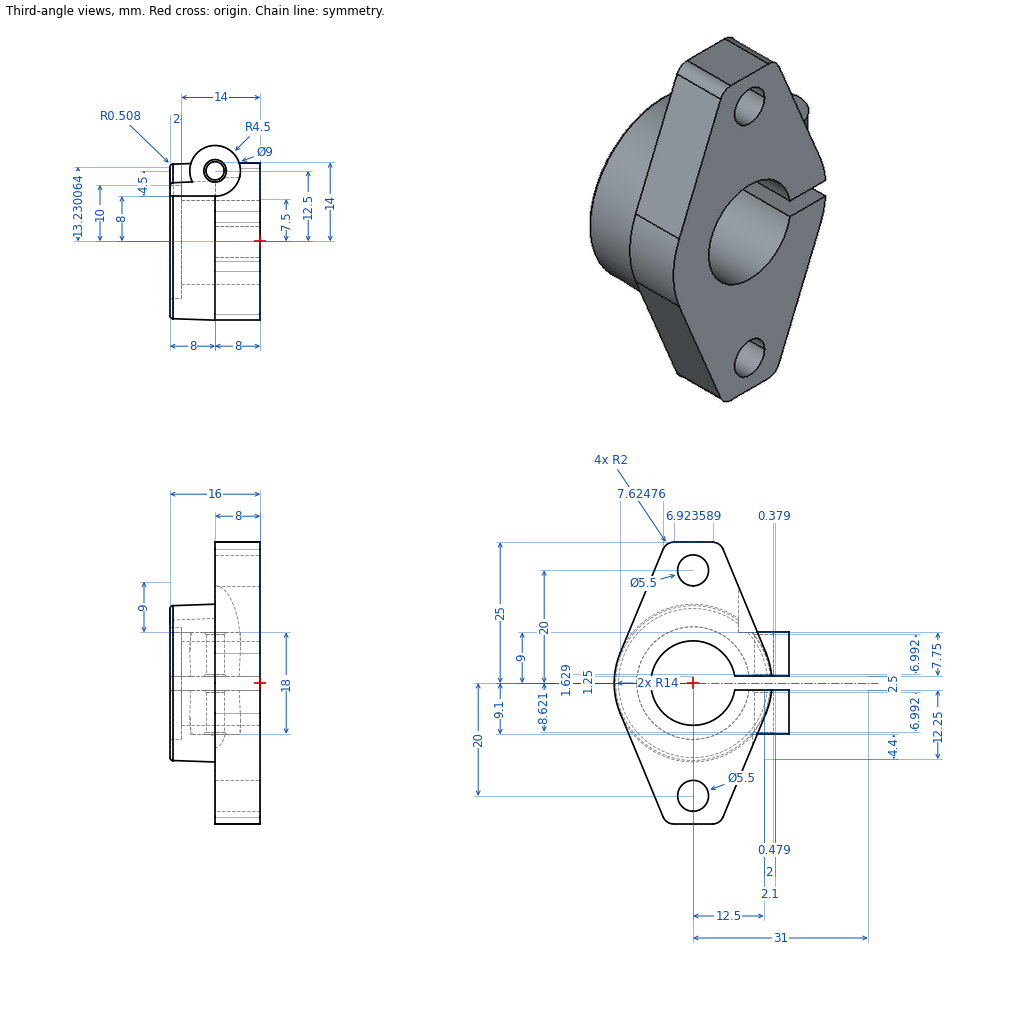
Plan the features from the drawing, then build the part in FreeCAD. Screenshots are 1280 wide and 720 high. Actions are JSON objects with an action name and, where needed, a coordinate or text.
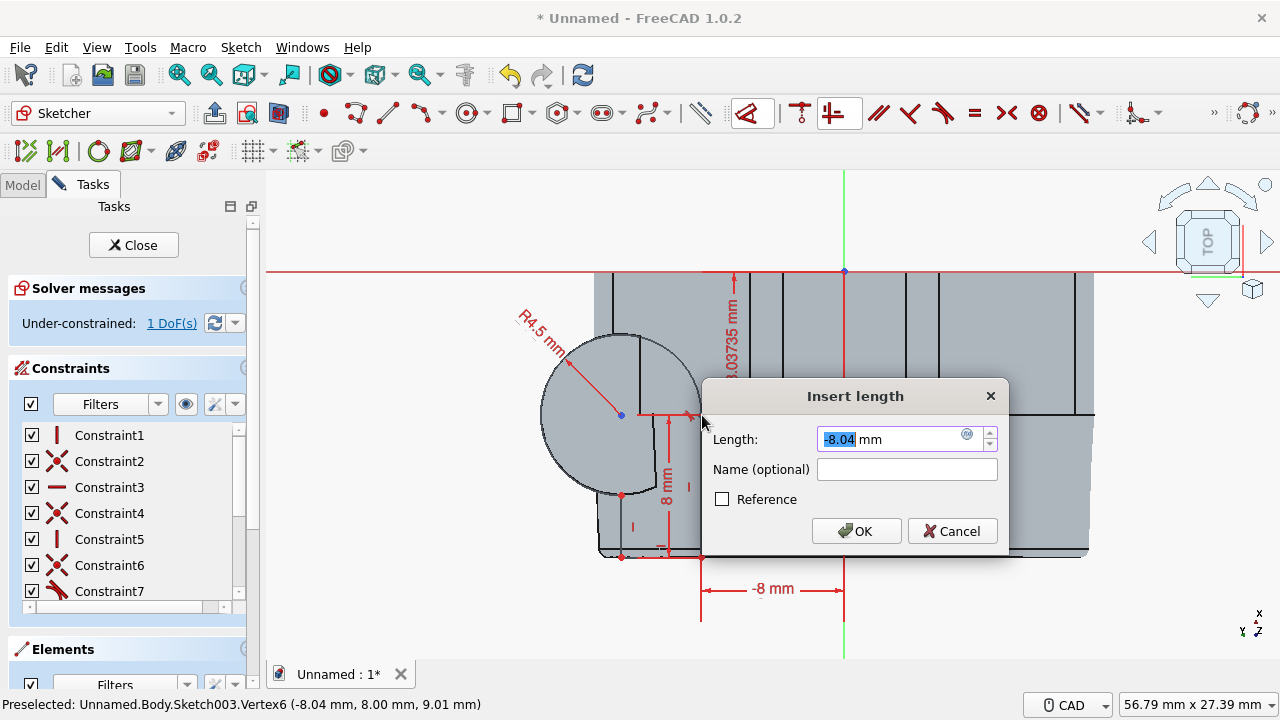
{"action": "type", "text": "-8"}
{"action": "key", "text": "Return"}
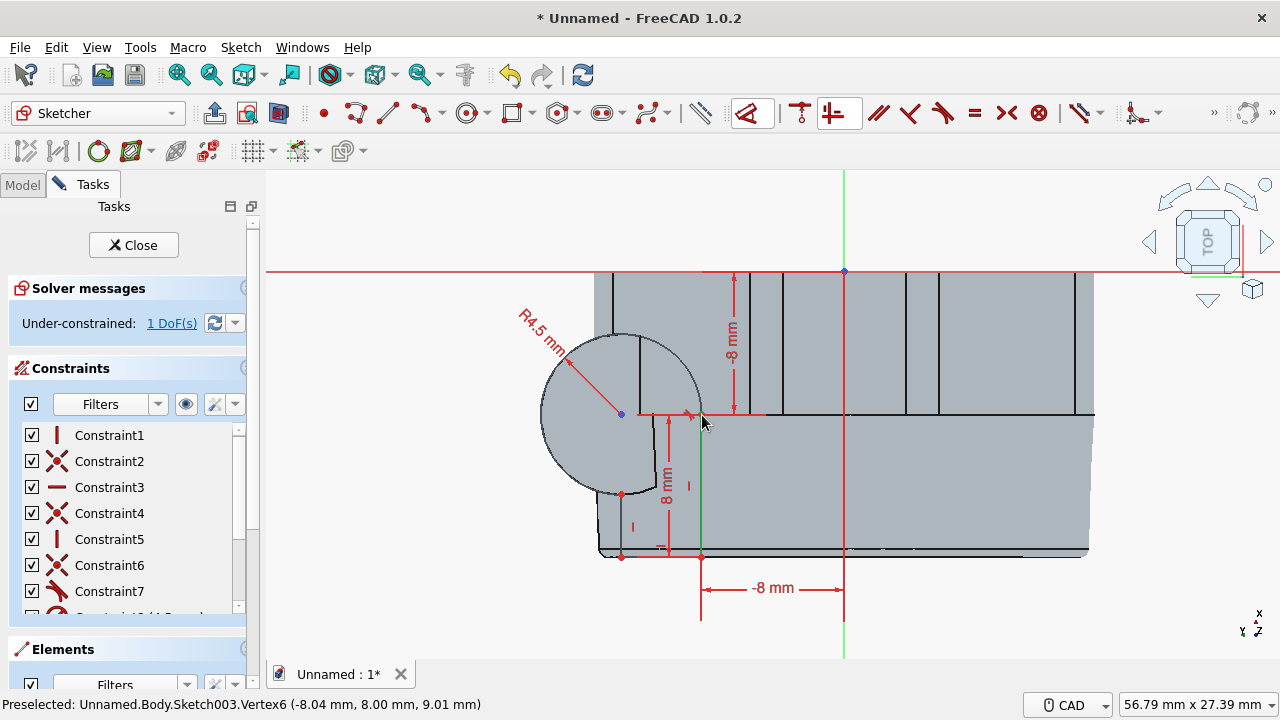
{"action": "left_click", "coordinate": [645, 557]}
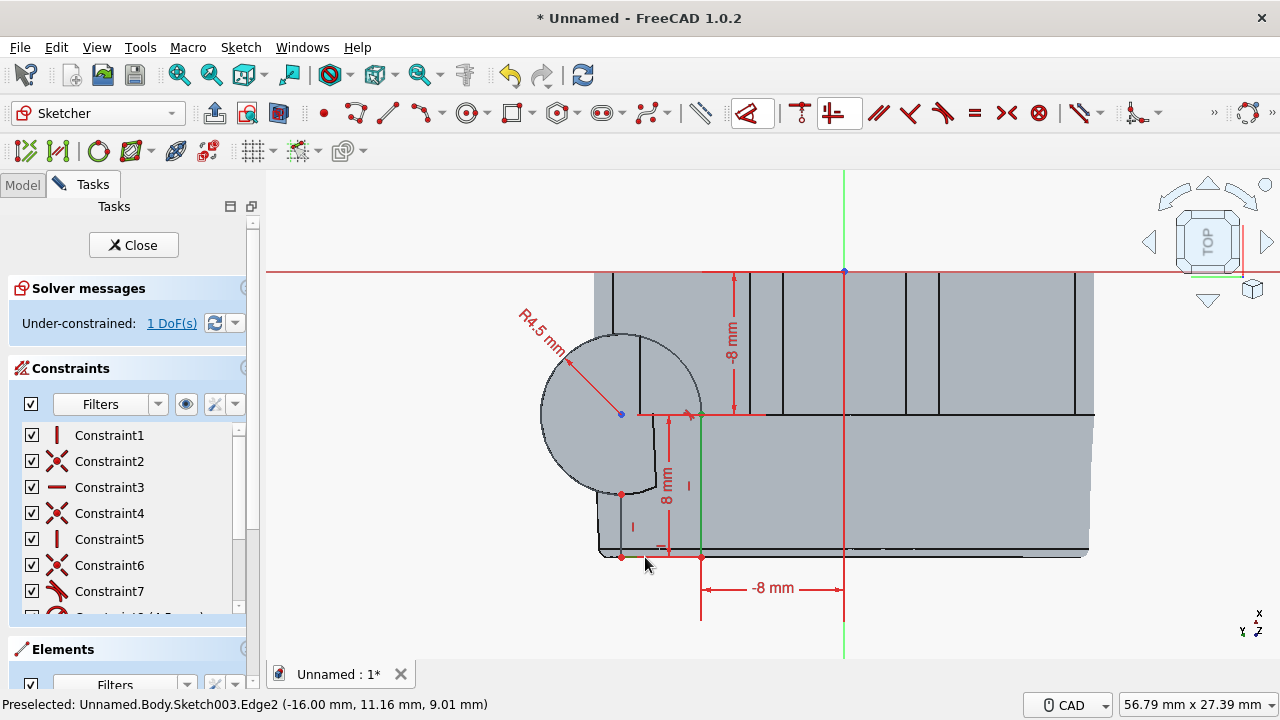
{"action": "left_click", "coordinate": [768, 114]}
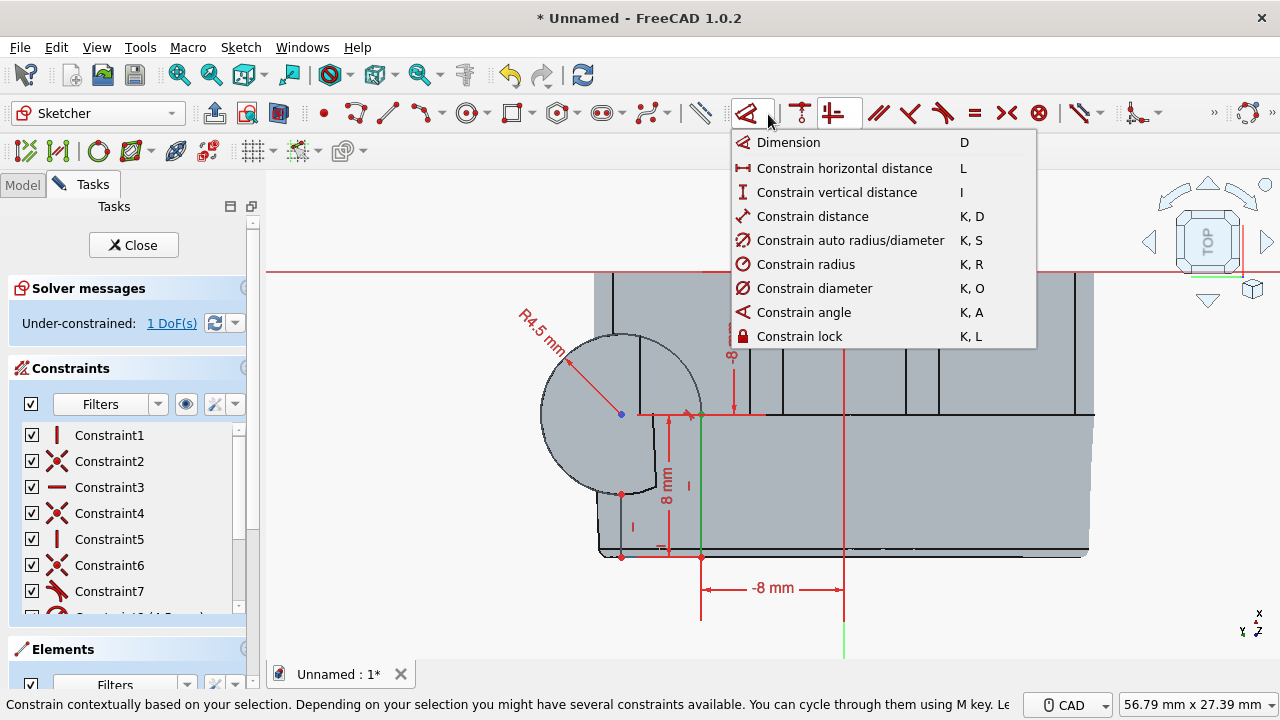
{"action": "left_click", "coordinate": [884, 168]}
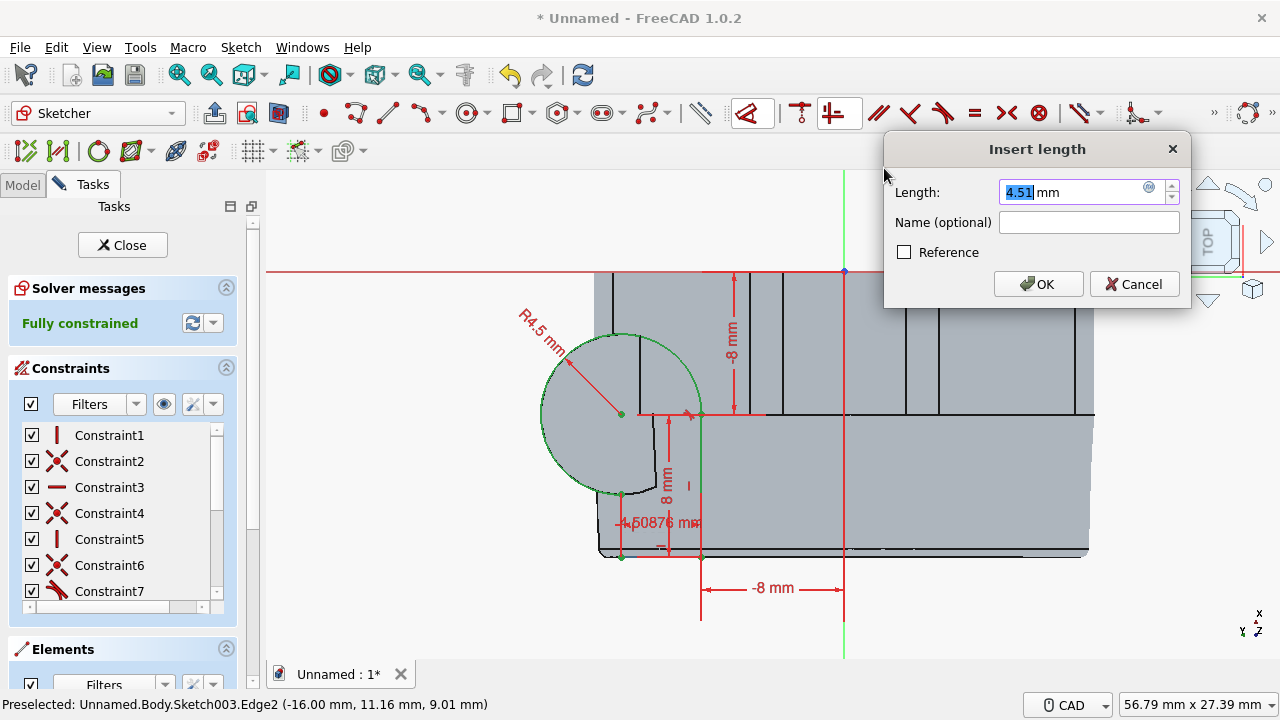
{"action": "type", "text": "4.5"}
{"action": "key", "text": "Return"}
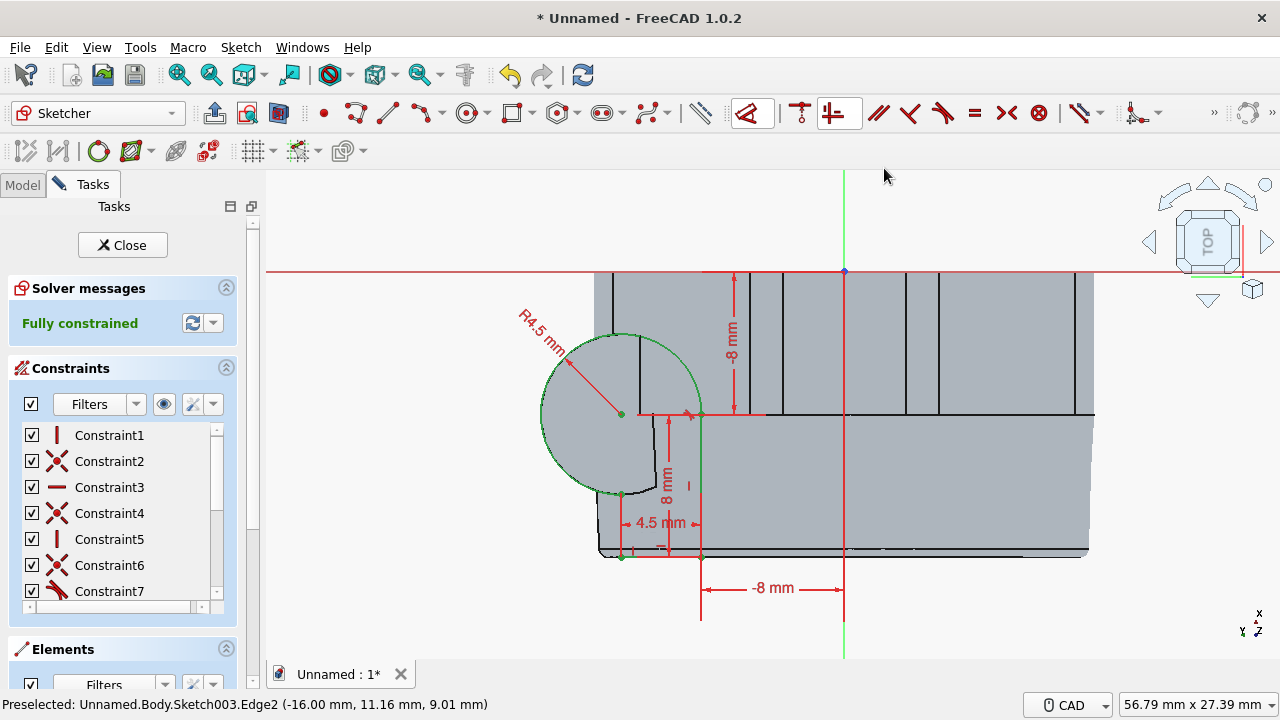
{"action": "left_click", "coordinate": [123, 245]}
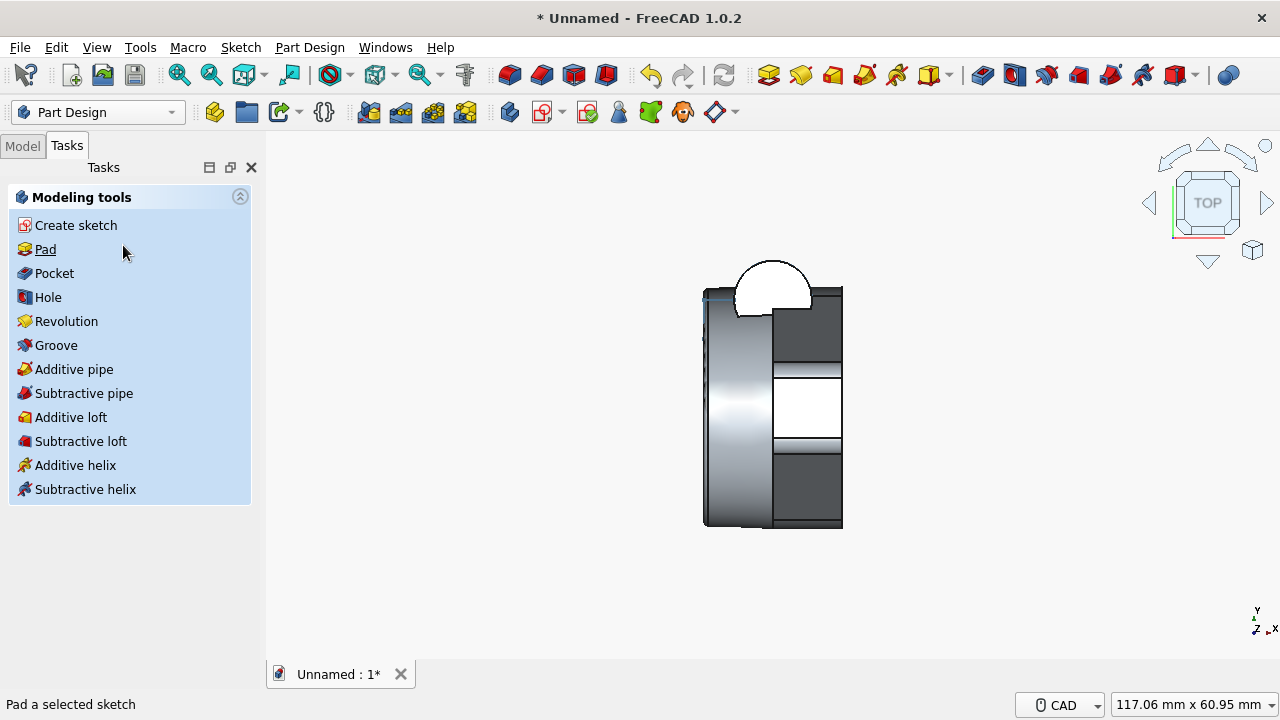
{"action": "left_click", "coordinate": [984, 76]}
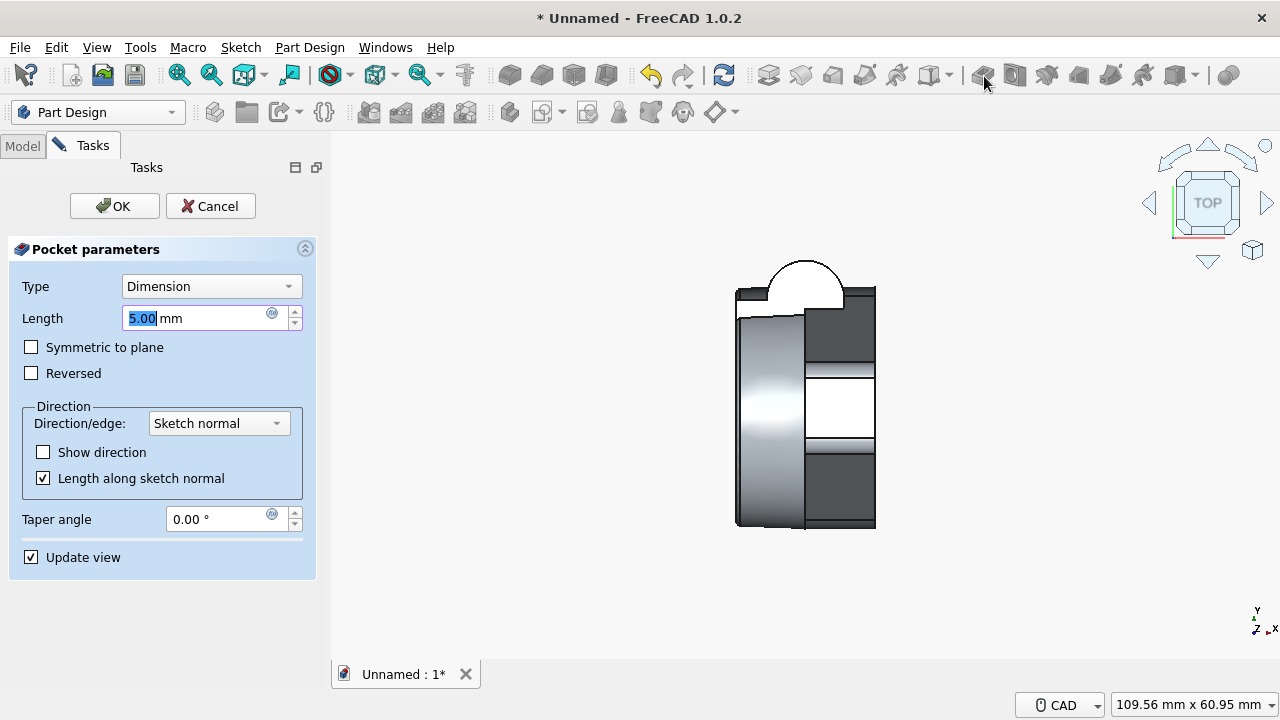
{"action": "type", "text": "9"}
{"action": "key", "text": "Tab"}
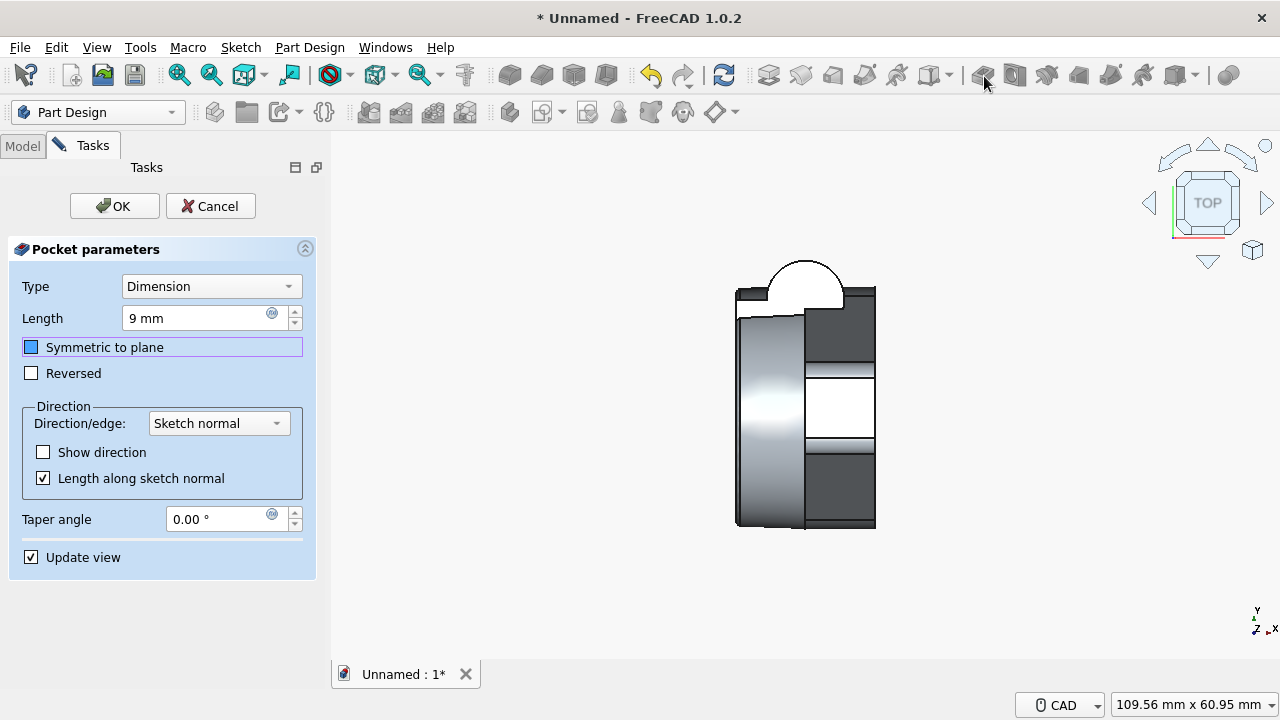
{"action": "left_click", "coordinate": [30, 373]}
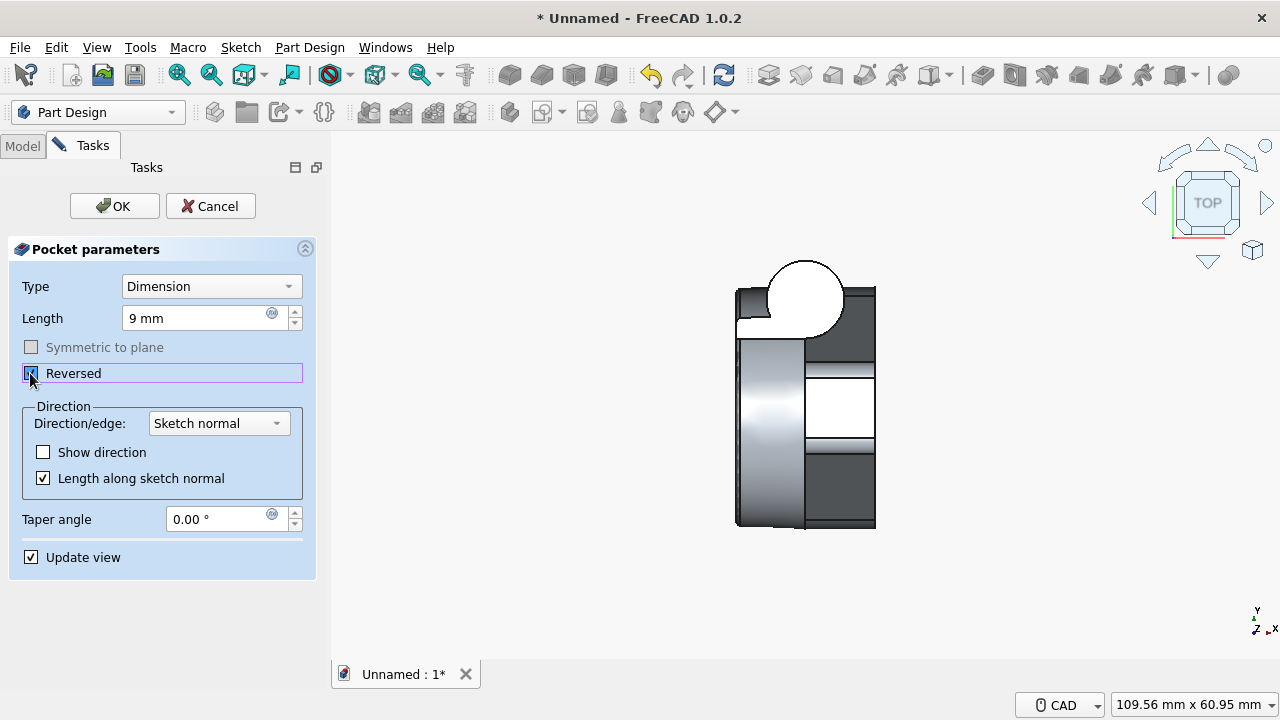
{"action": "left_click", "coordinate": [115, 206]}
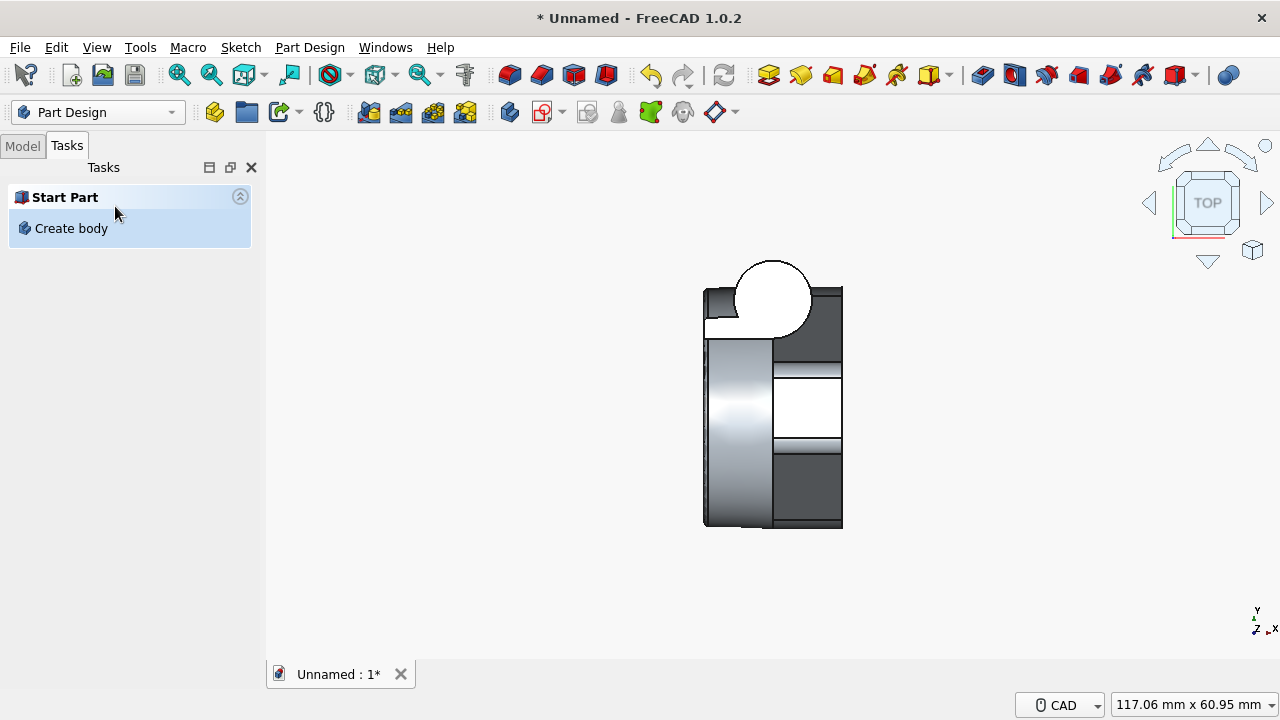
{"action": "key", "text": "0"}